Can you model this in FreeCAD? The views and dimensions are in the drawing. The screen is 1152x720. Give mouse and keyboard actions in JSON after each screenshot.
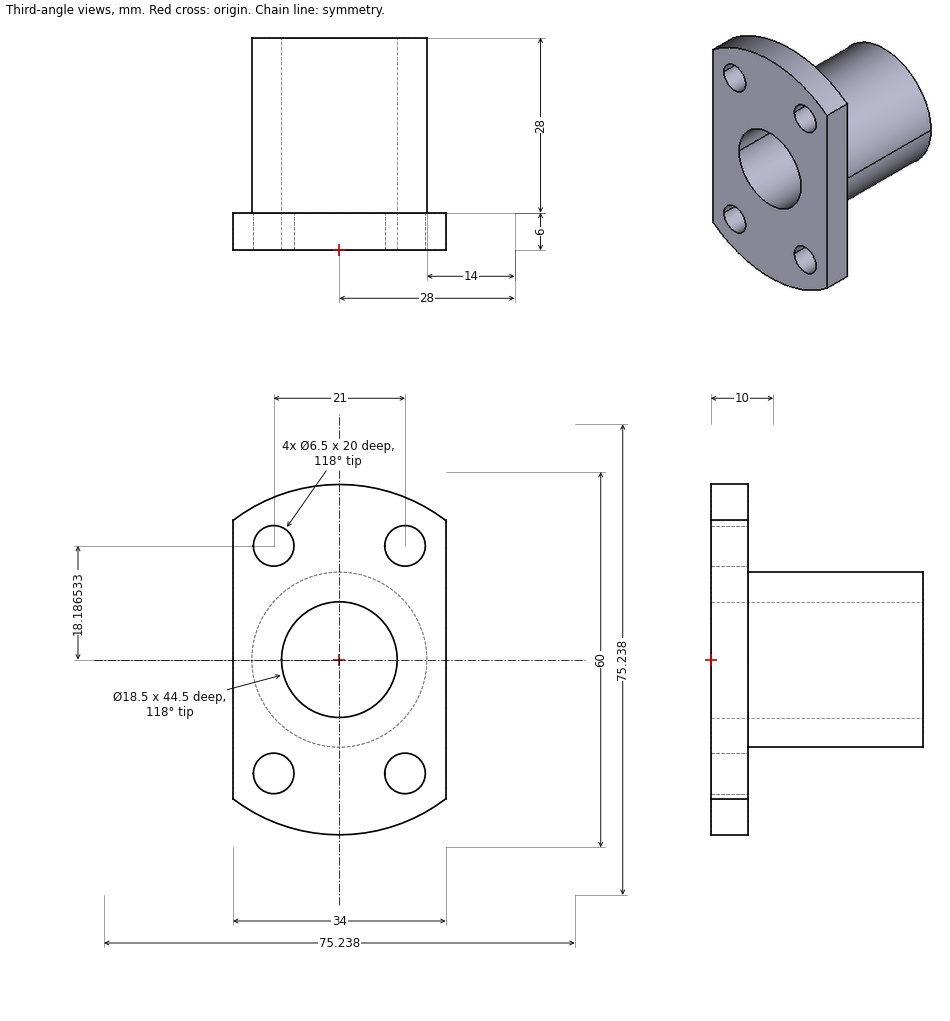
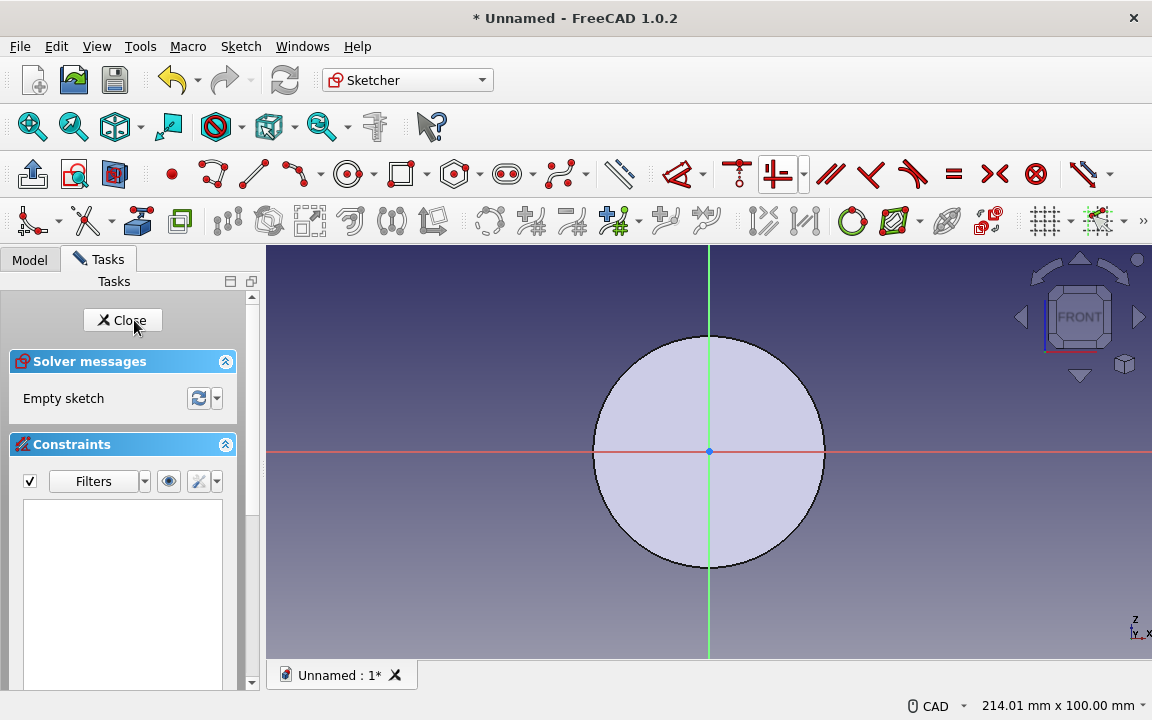
{"action": "scroll", "coordinate": [331, 452], "scroll_direction": "down", "scroll_amount": 1}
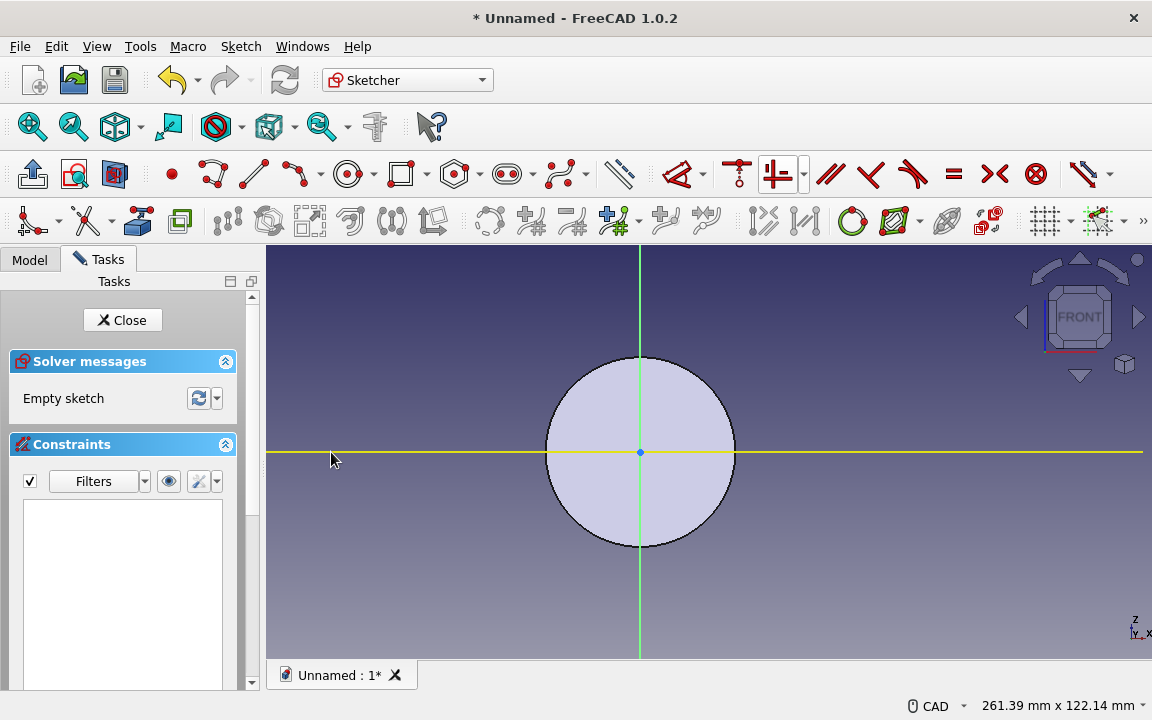
{"action": "left_click", "coordinate": [426, 174]}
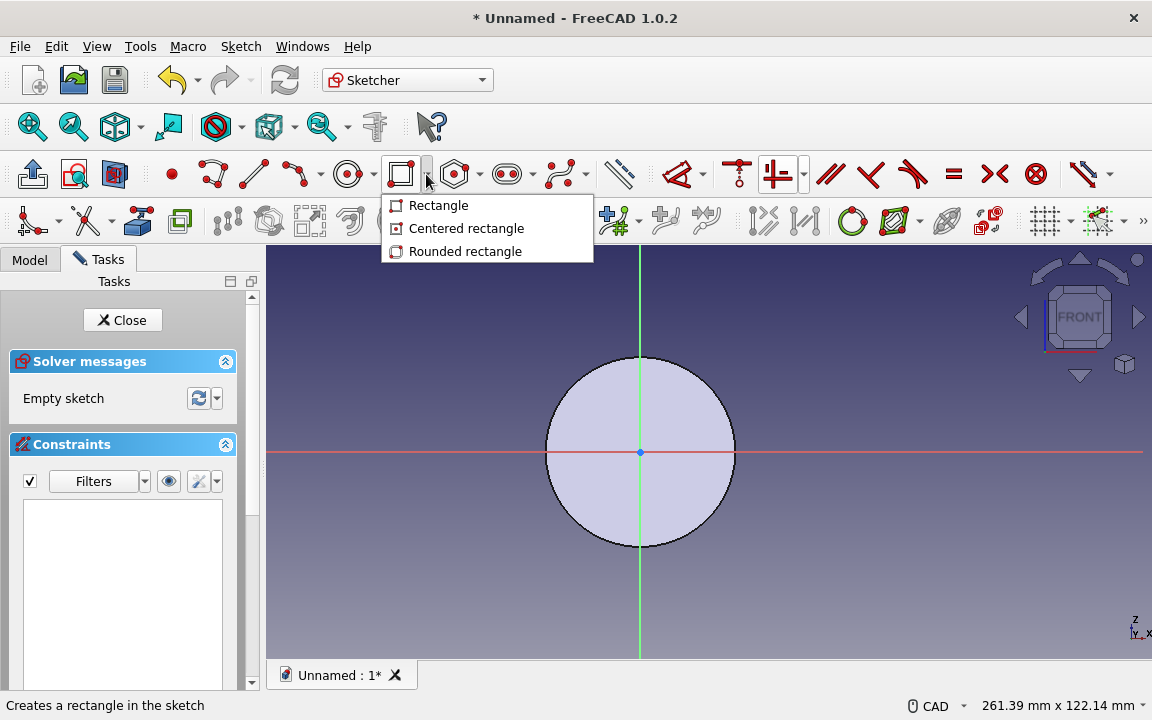
{"action": "left_click", "coordinate": [488, 228]}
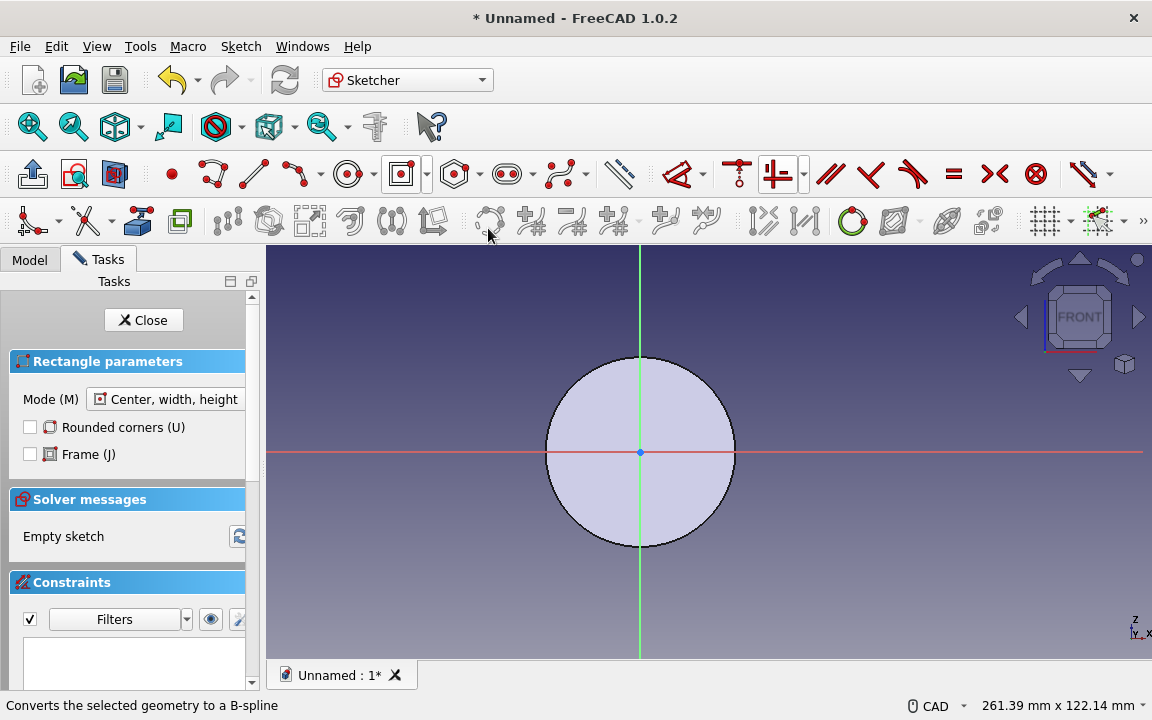
{"action": "left_click", "coordinate": [640, 452]}
{"action": "mouse_move", "coordinate": [768, 325]}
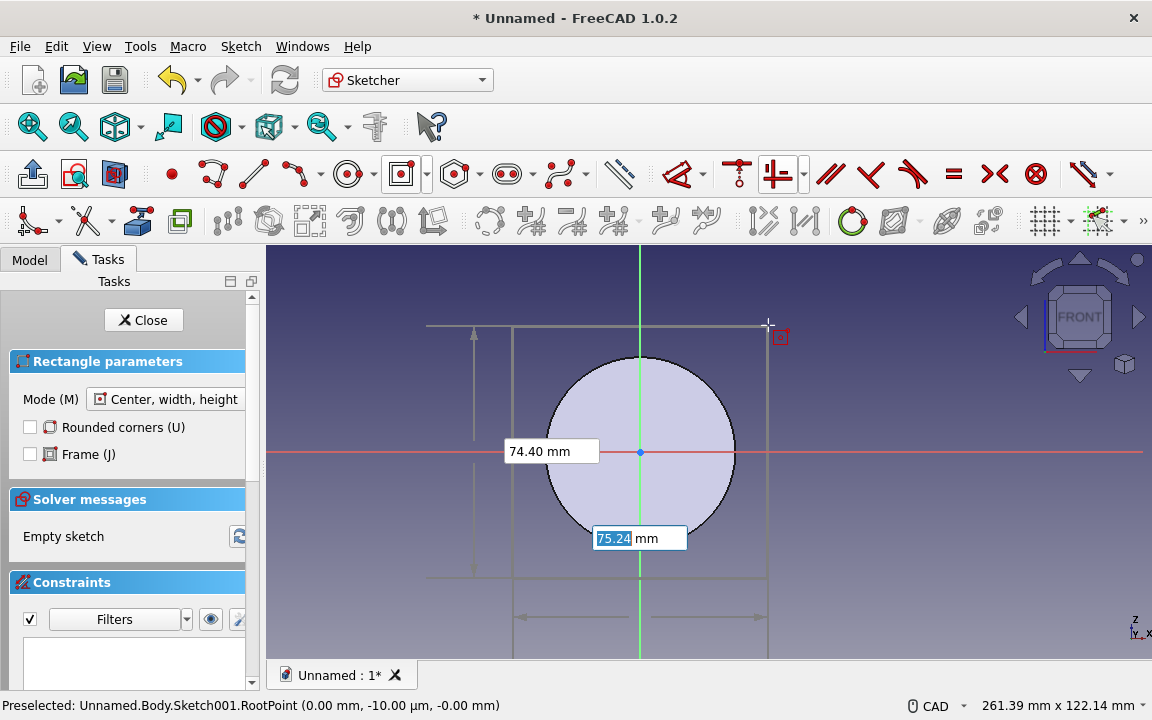
{"action": "type", "text": "75.238"}
{"action": "key", "text": "Tab"}
{"action": "type", "text": "75.238"}
{"action": "key", "text": "Return"}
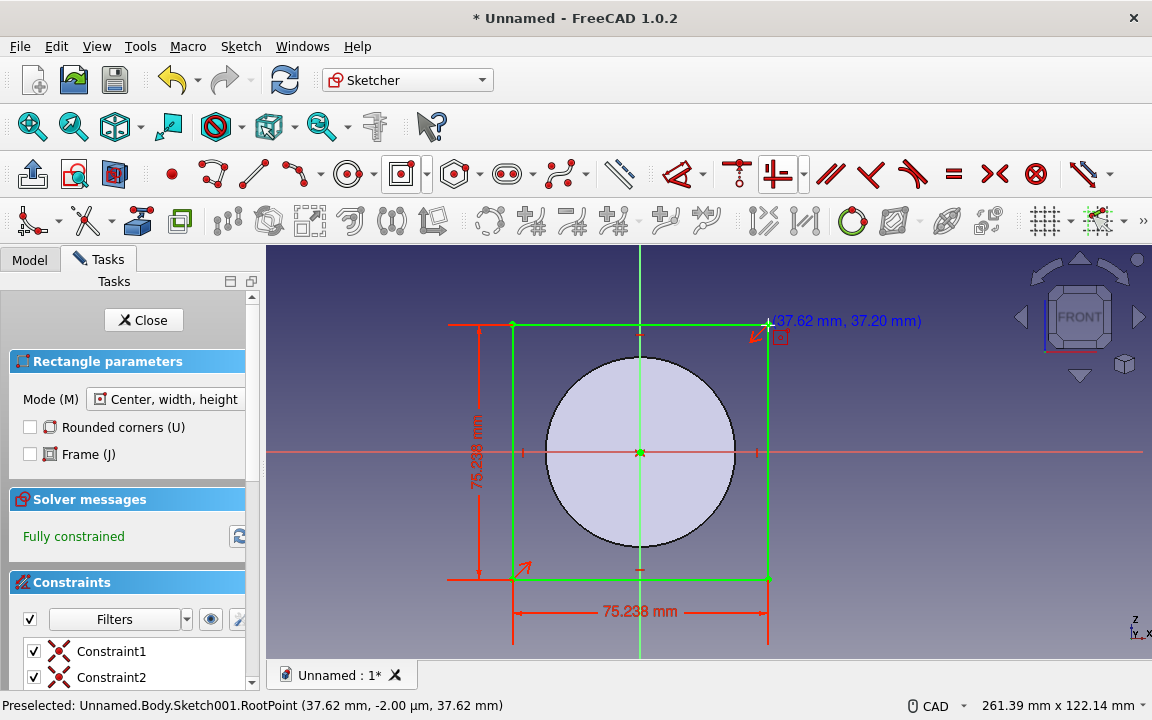
{"action": "left_click", "coordinate": [640, 452]}
{"action": "mouse_move", "coordinate": [698, 350]}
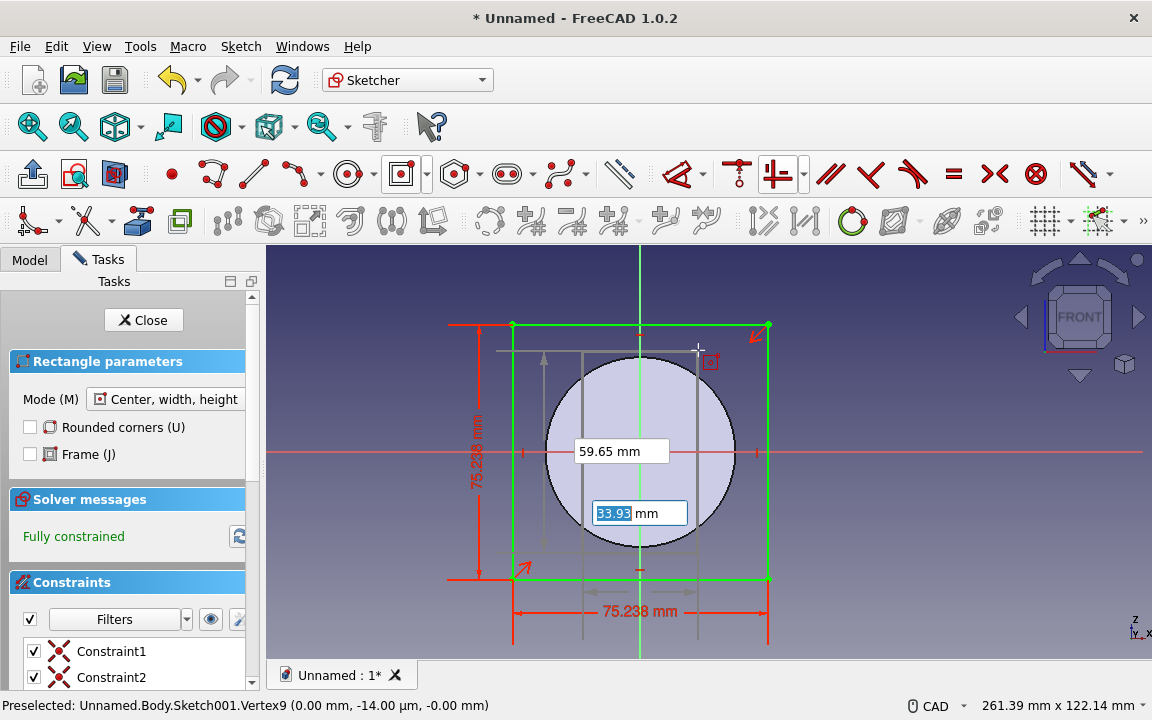
{"action": "type", "text": "34"}
{"action": "key", "text": "Tab"}
{"action": "type", "text": "60"}
{"action": "key", "text": "Return"}
{"action": "key", "text": "Escape"}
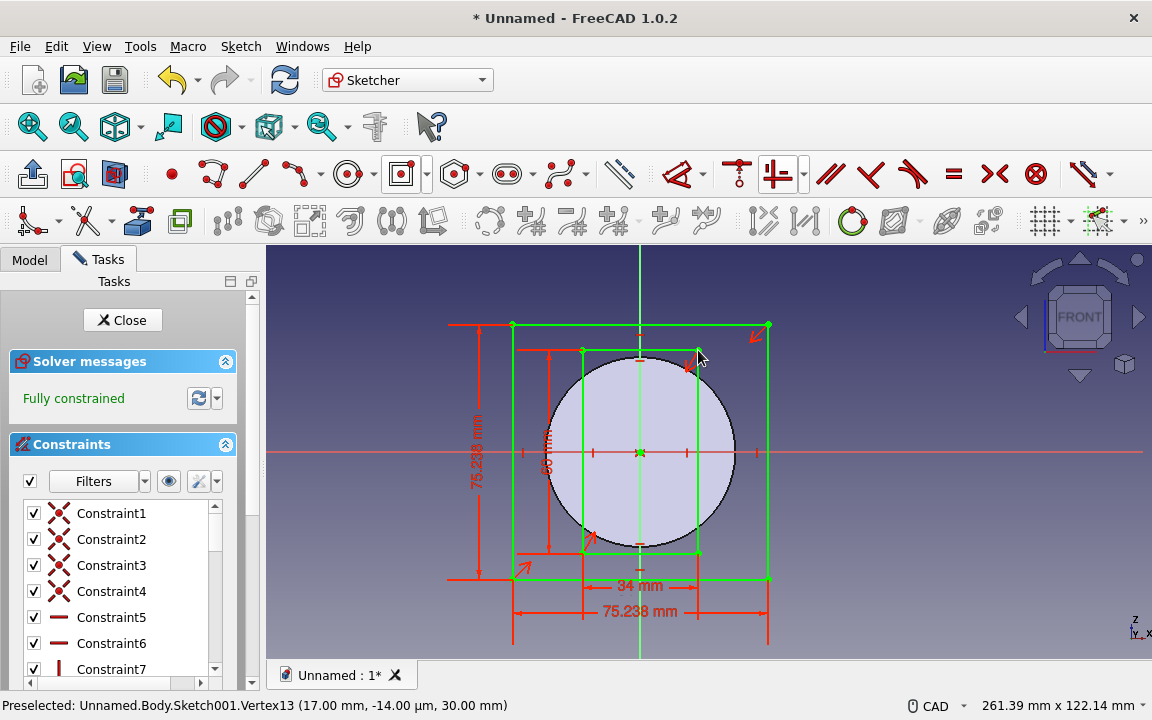
{"action": "left_click", "coordinate": [123, 320]}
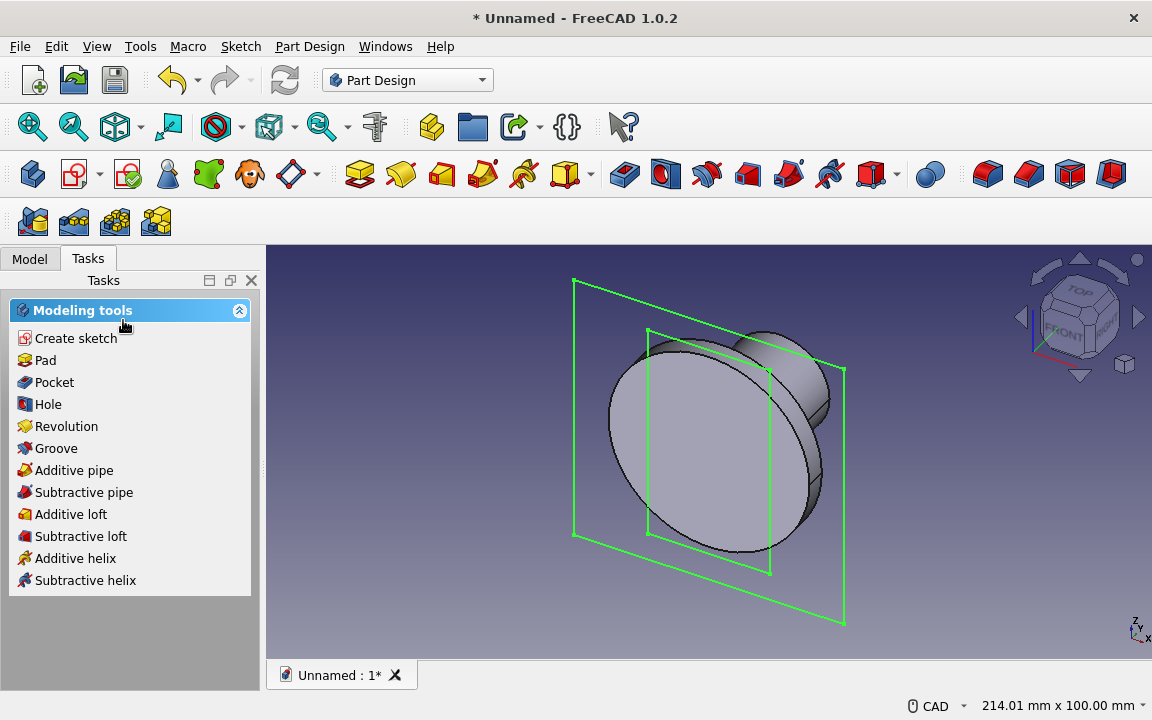
{"action": "left_click", "coordinate": [625, 174]}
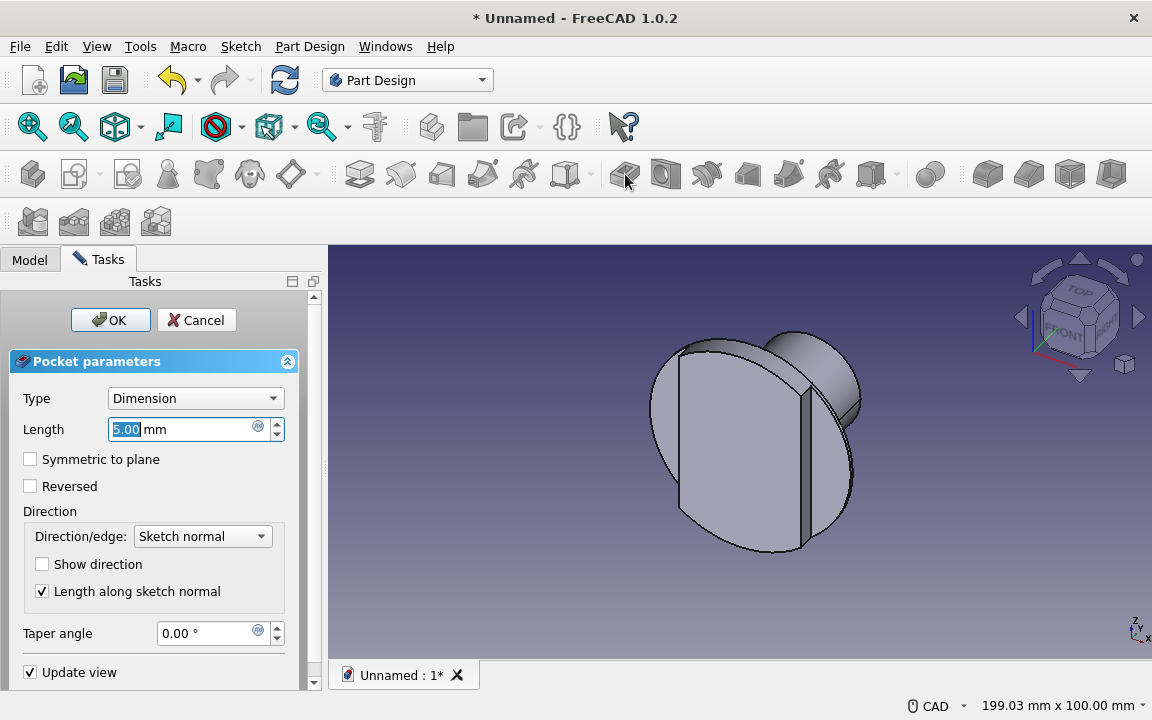
{"action": "type", "text": "10"}
{"action": "key", "text": "Tab"}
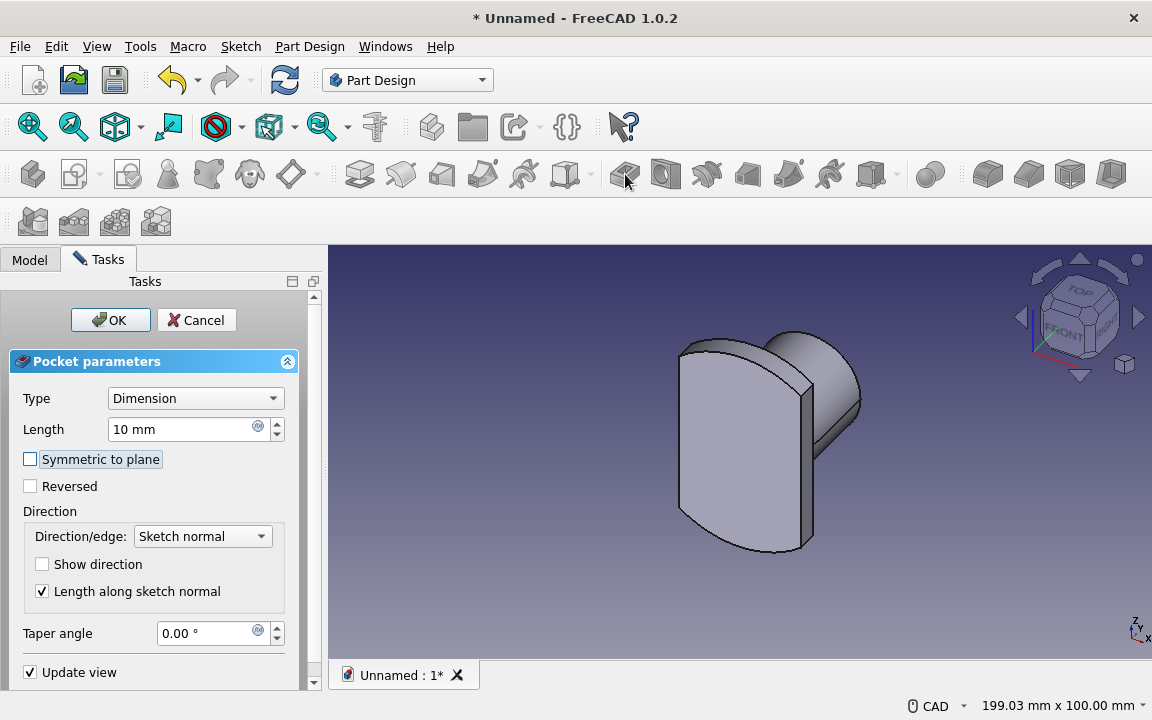
{"action": "left_click", "coordinate": [111, 320]}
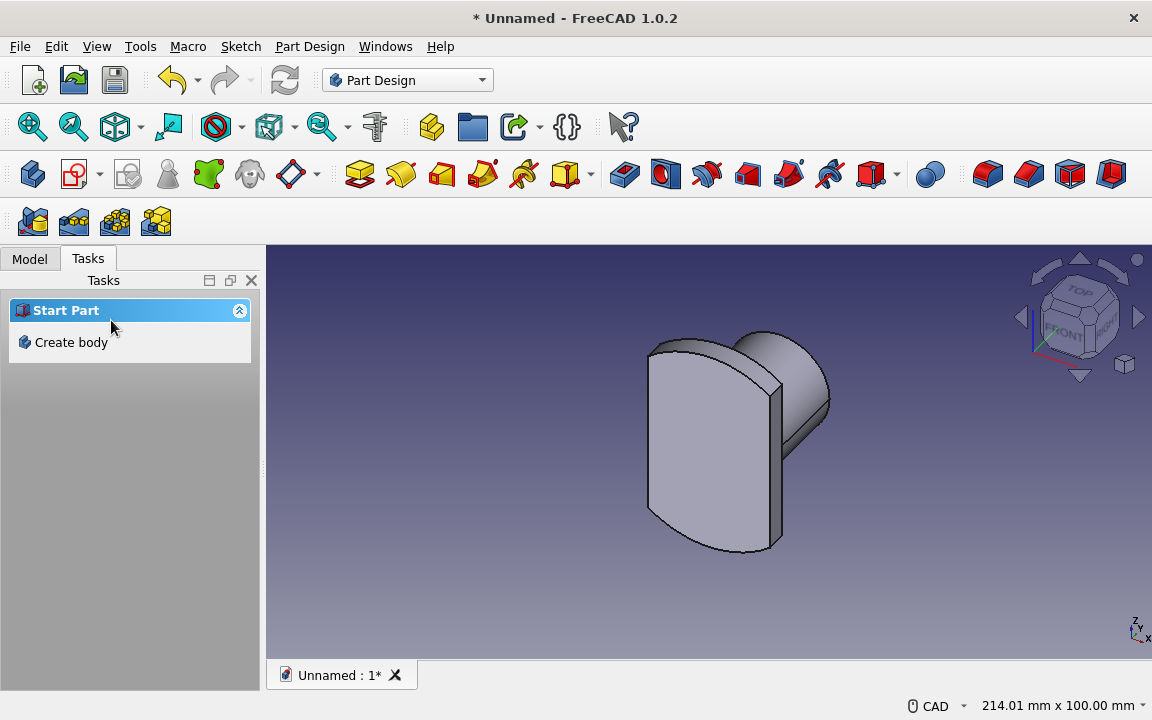
{"action": "left_click", "coordinate": [74, 174]}